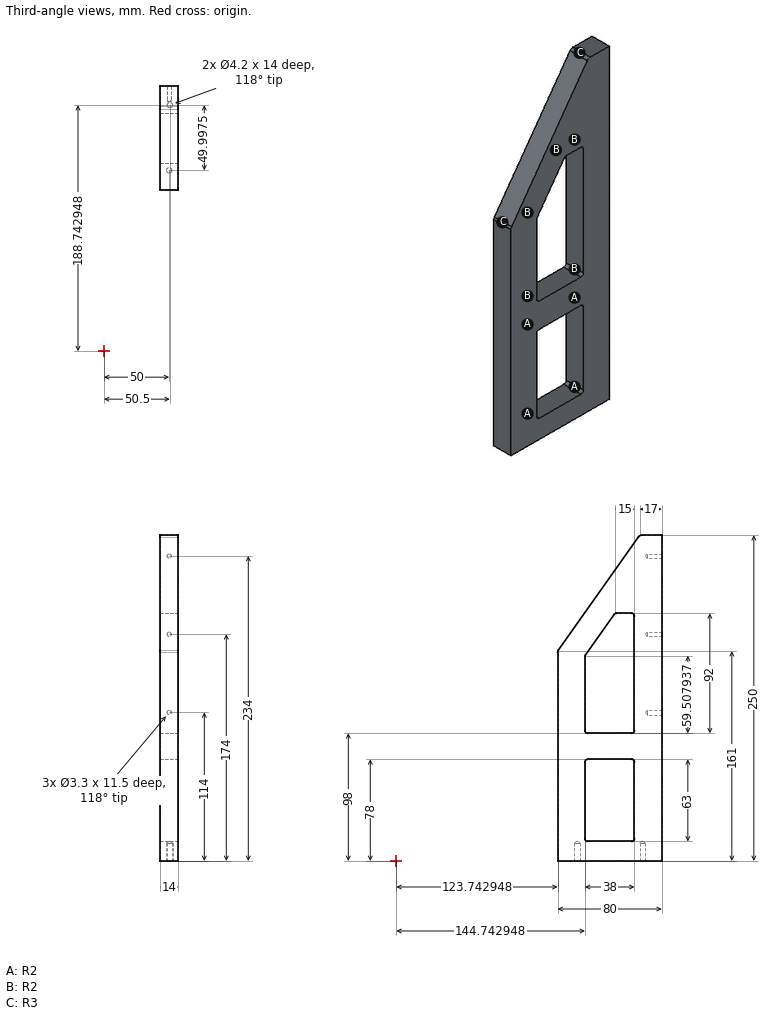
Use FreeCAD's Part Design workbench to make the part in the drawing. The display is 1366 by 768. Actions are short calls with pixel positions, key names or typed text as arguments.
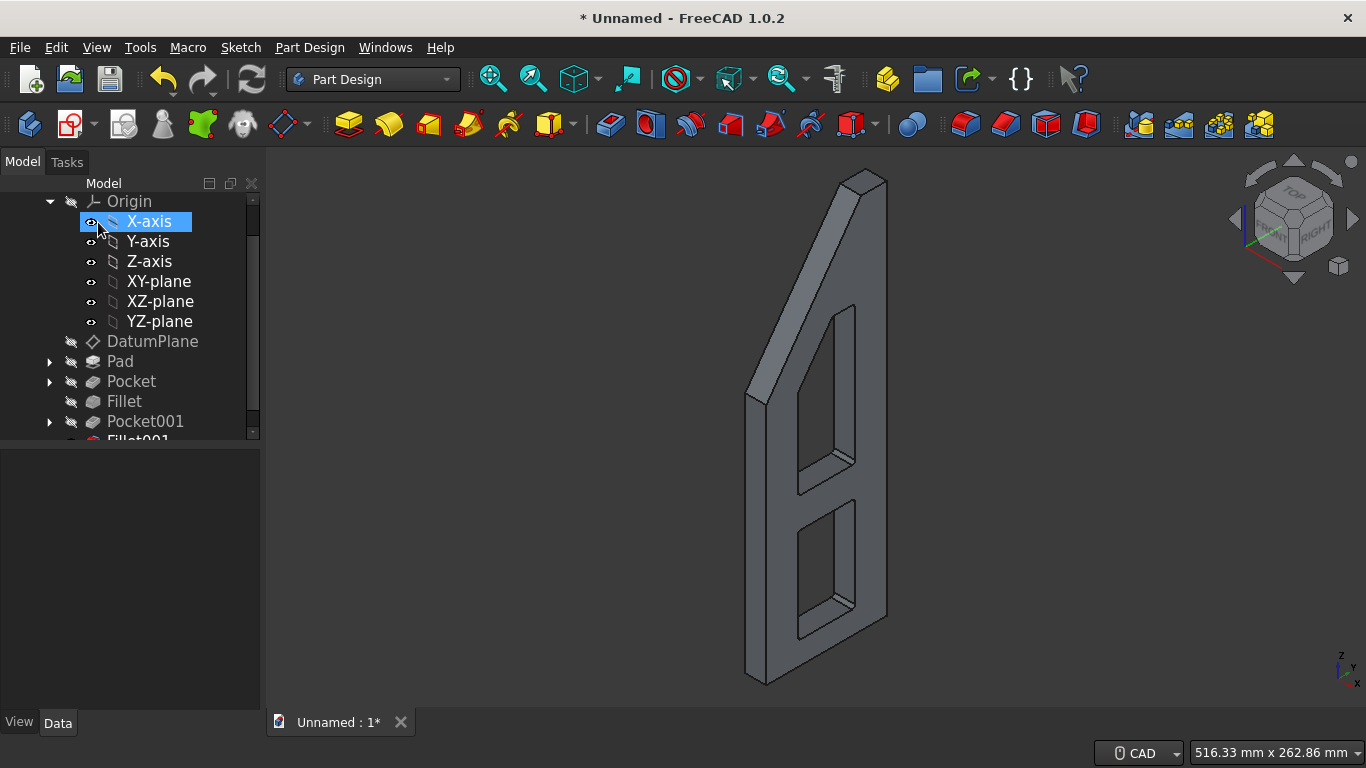
click(70, 124)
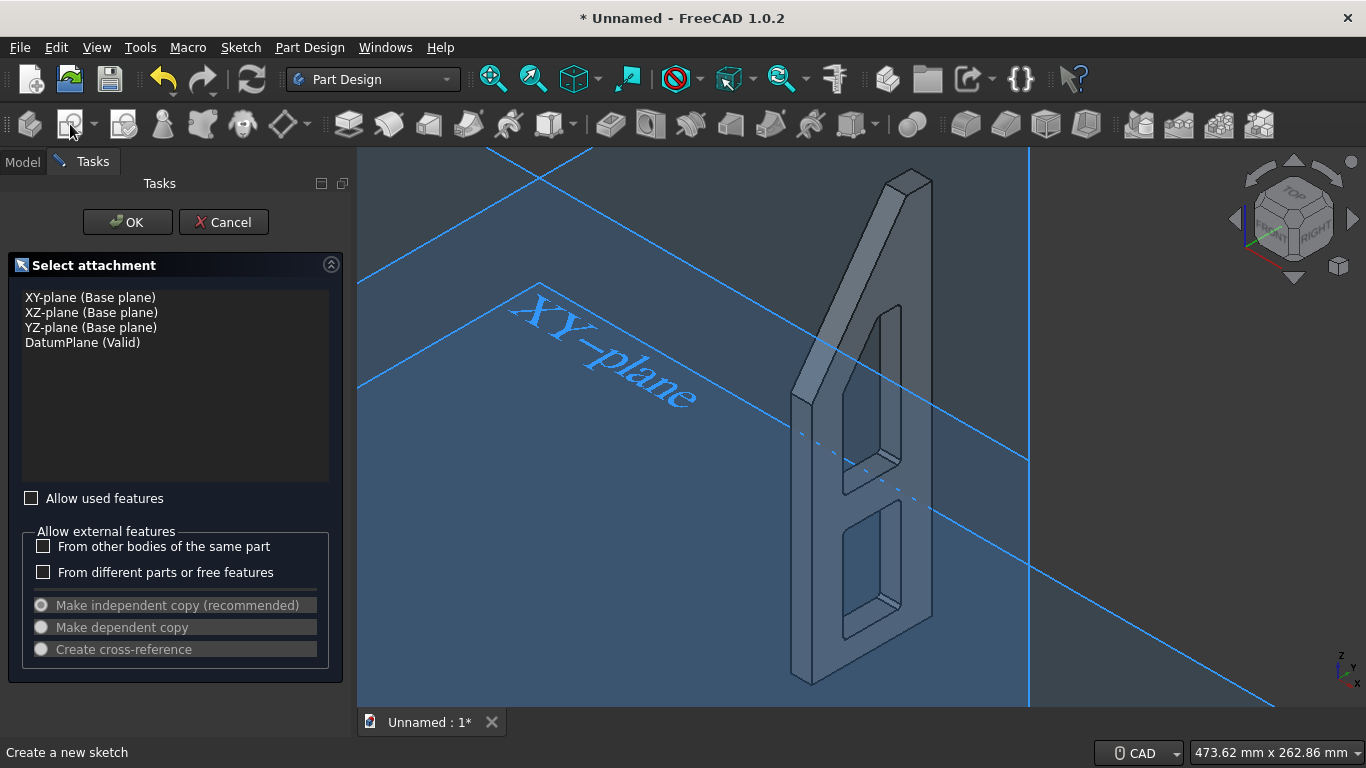
click(82, 298)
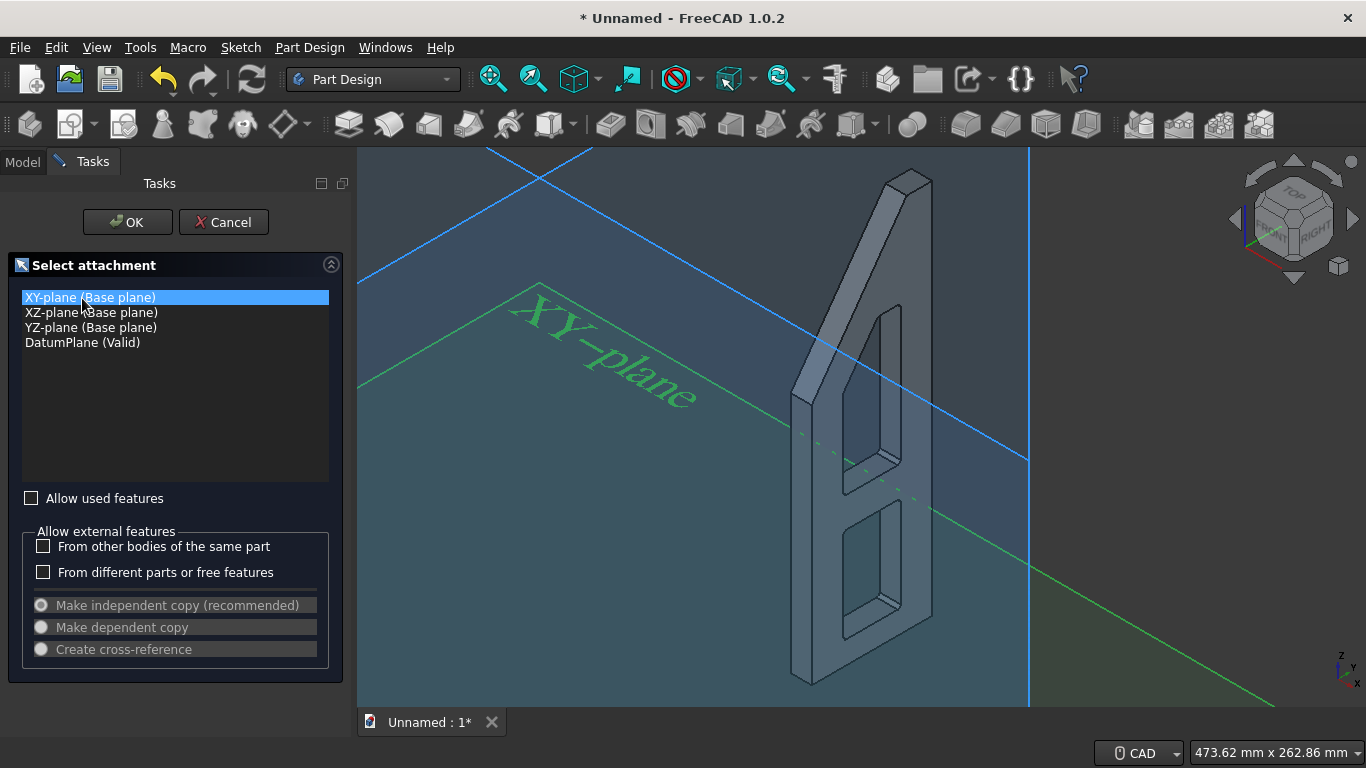
click(128, 222)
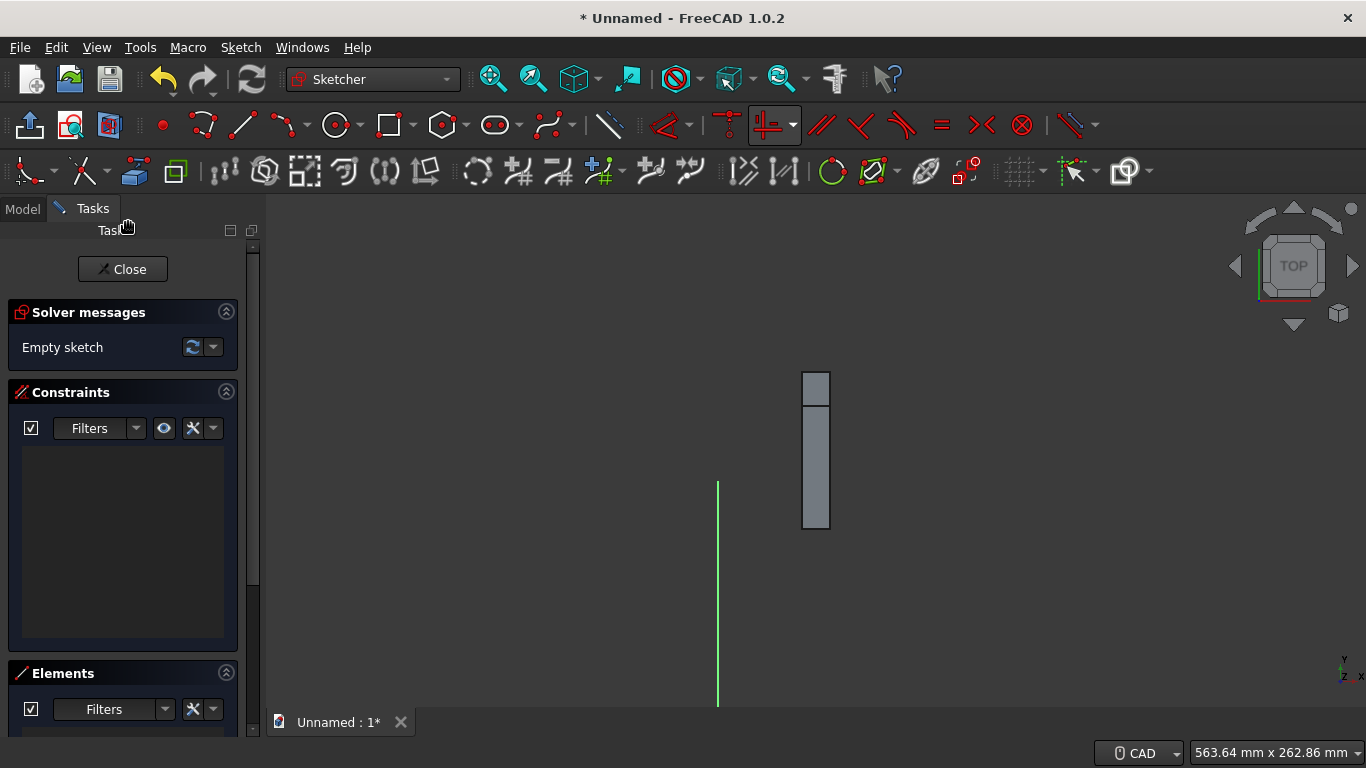
click(110, 126)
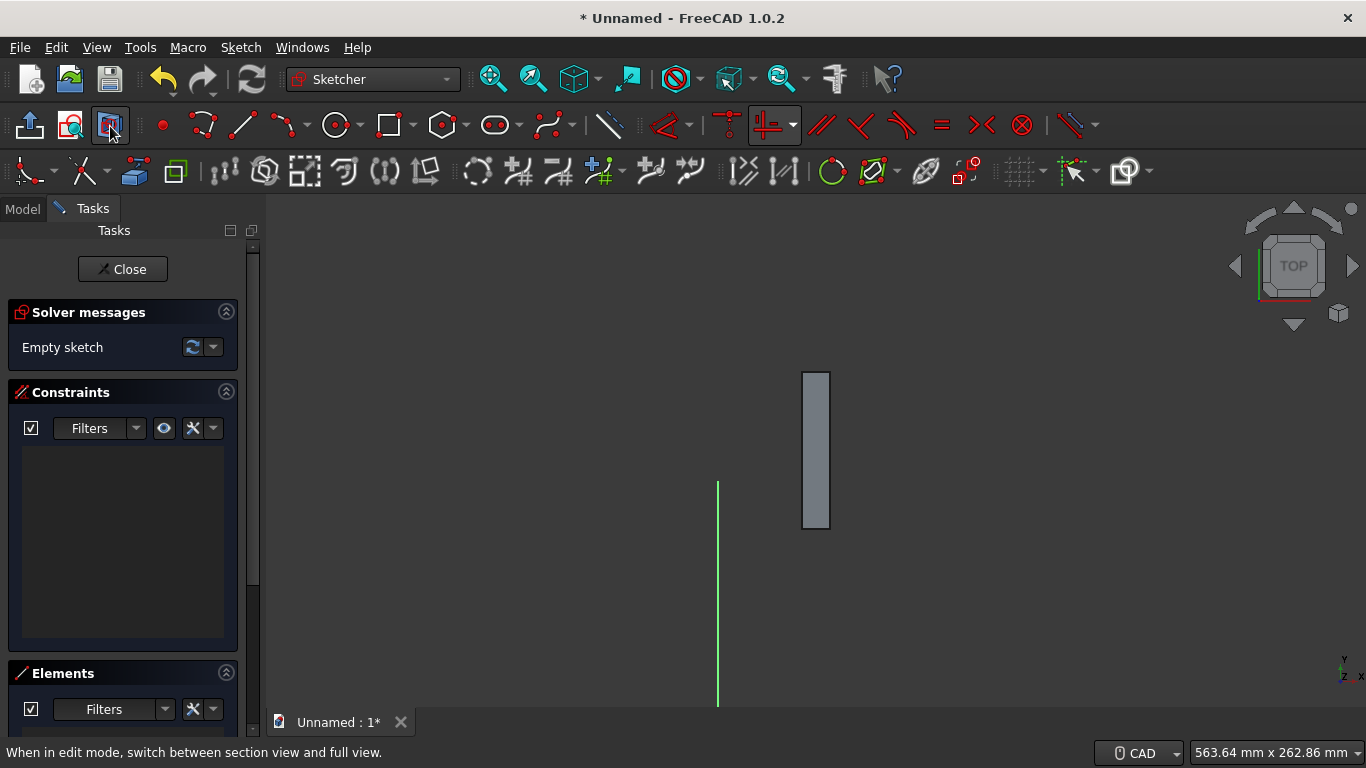
scroll(846, 450, up, 6)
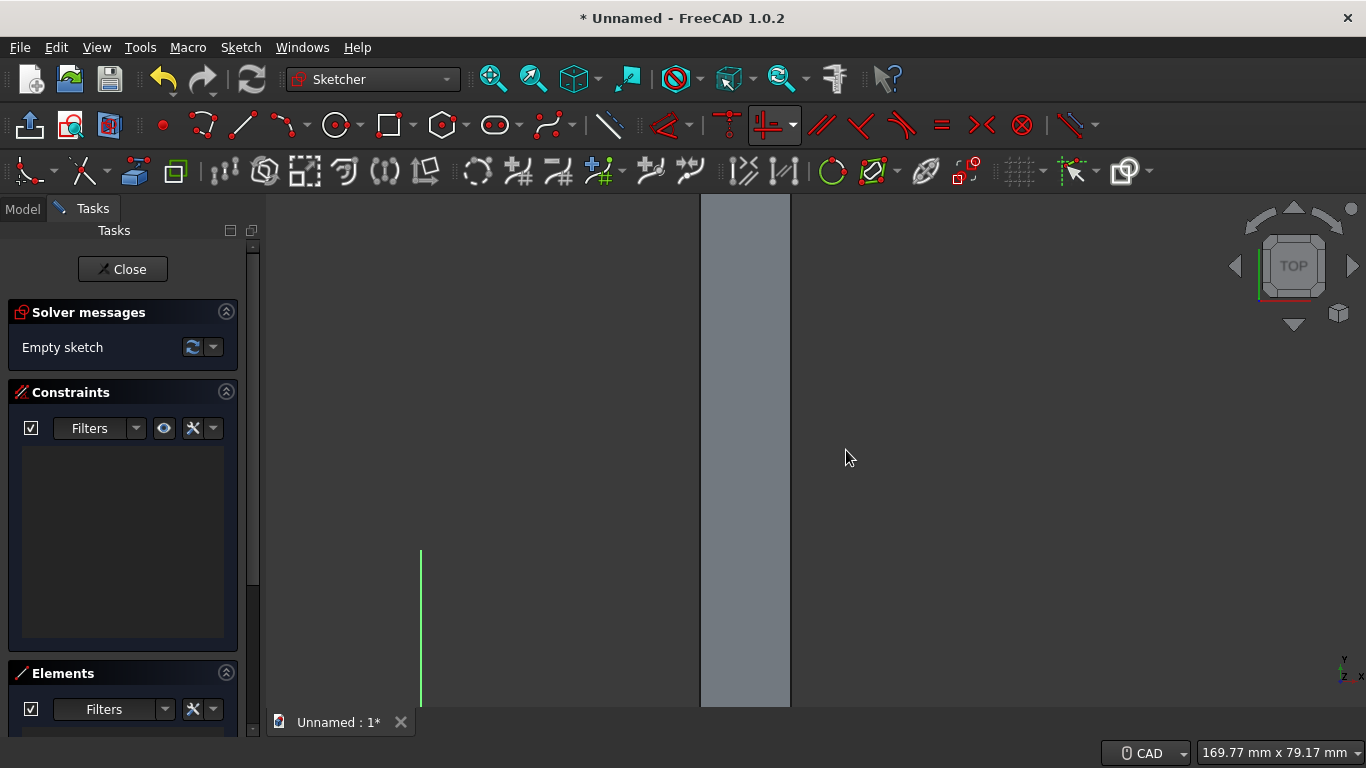
click(336, 126)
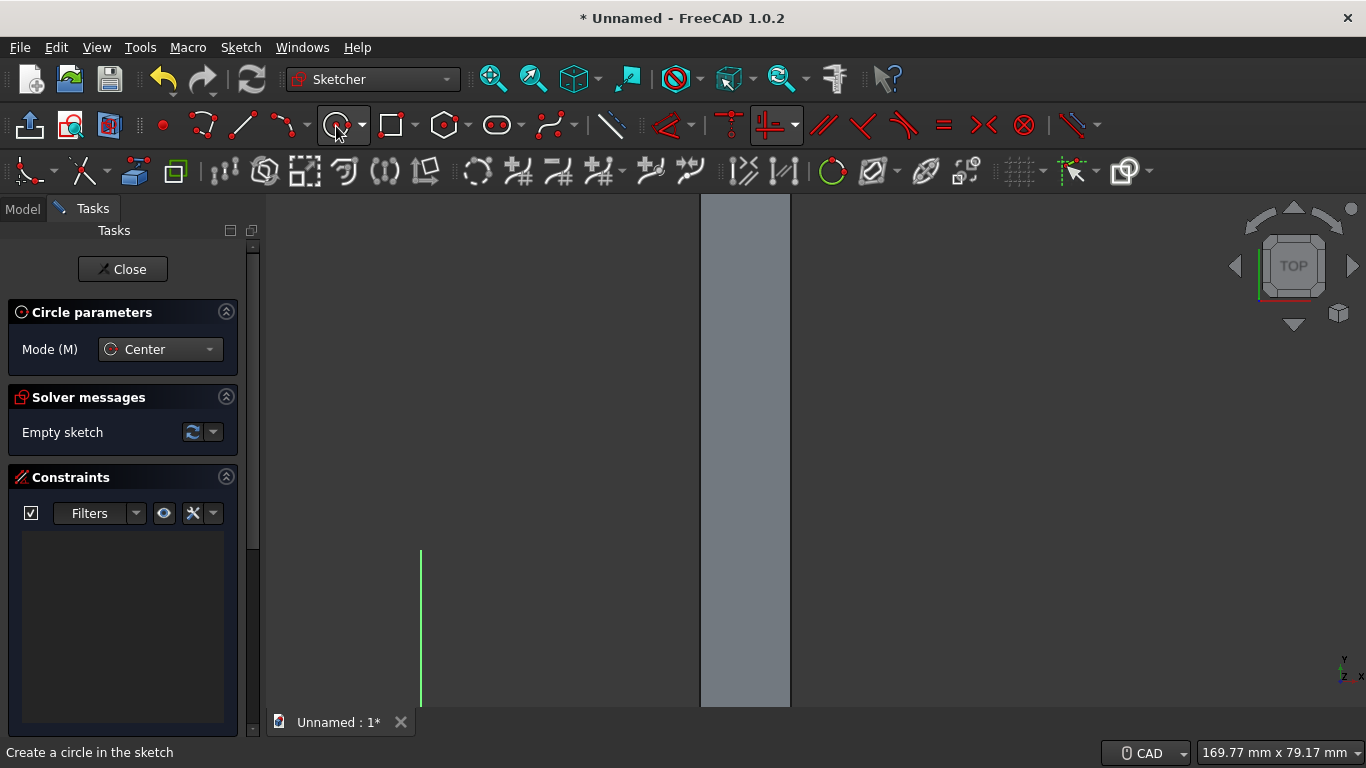
scroll(748, 289, up, 3)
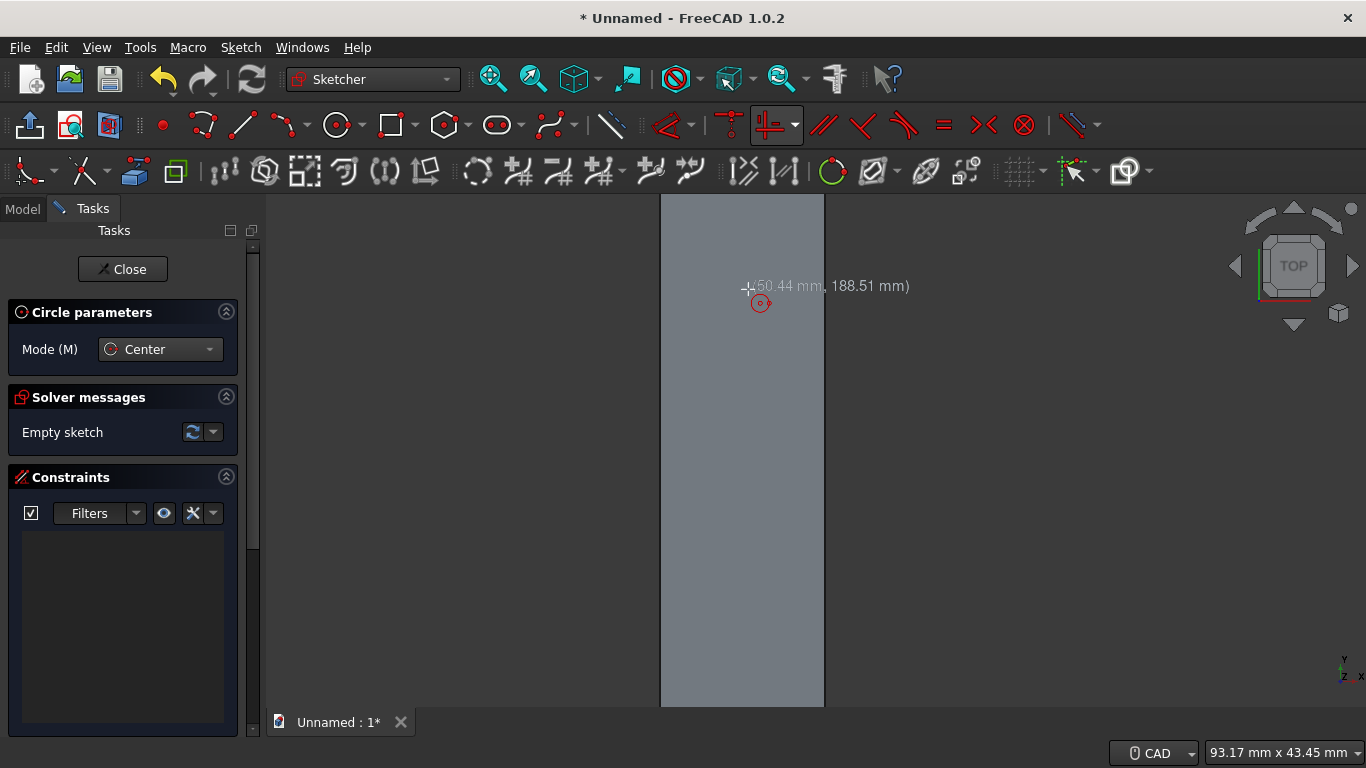
click(748, 288)
click(766, 270)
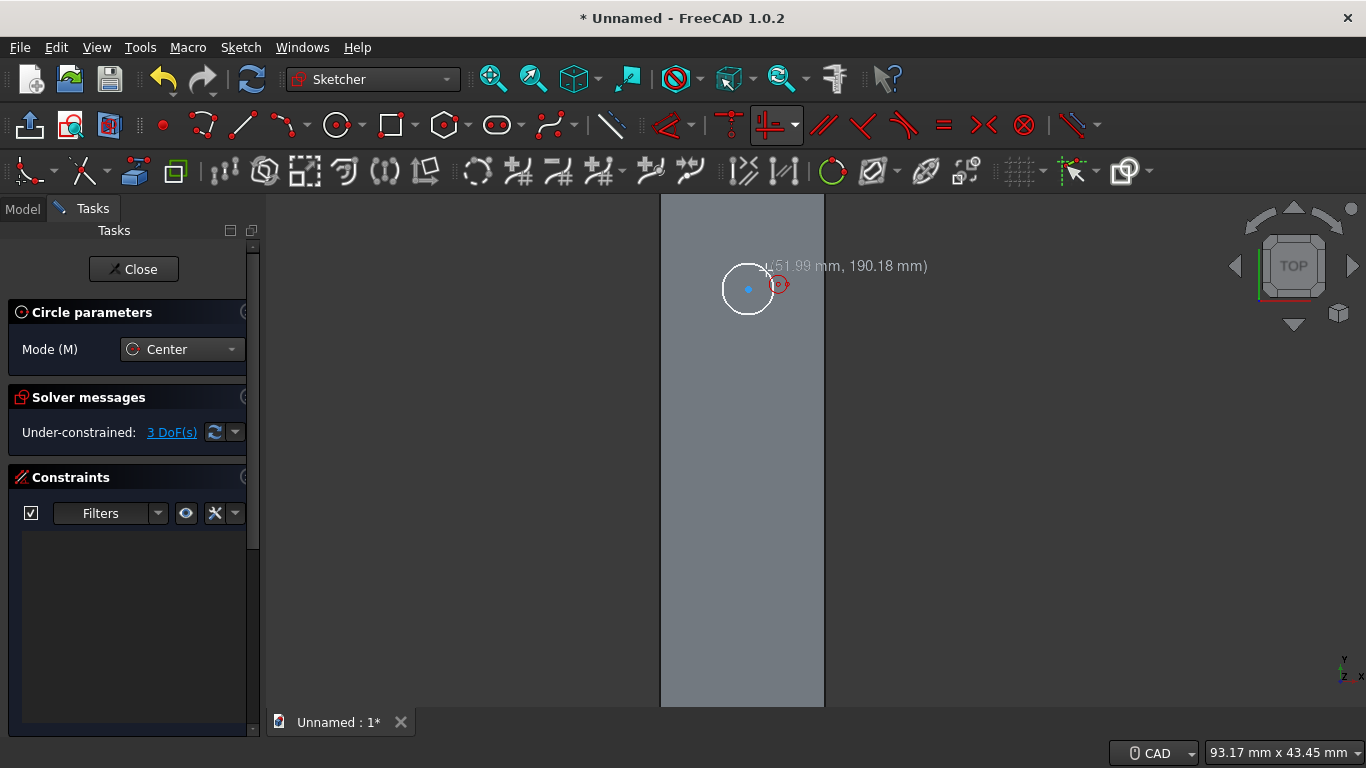
scroll(750, 289, down, 3)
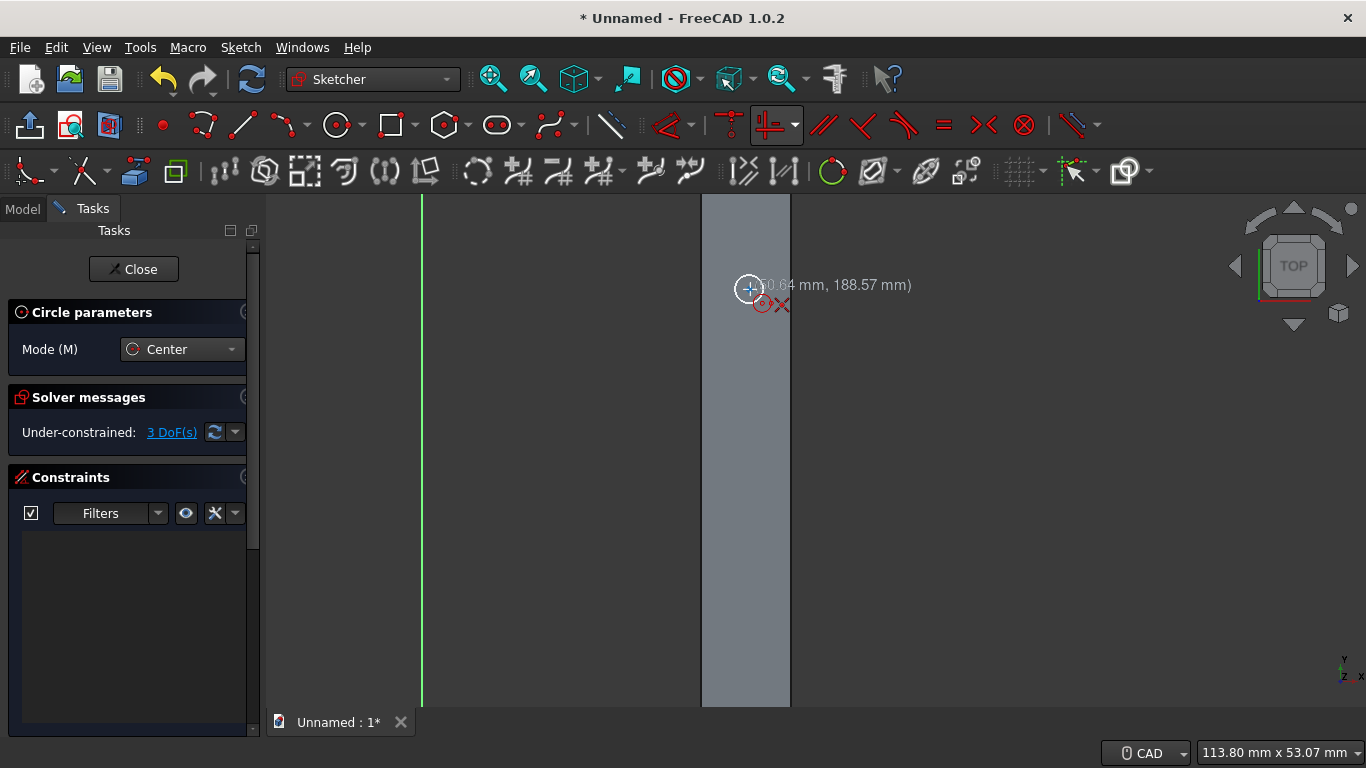
scroll(746, 612, up, 3)